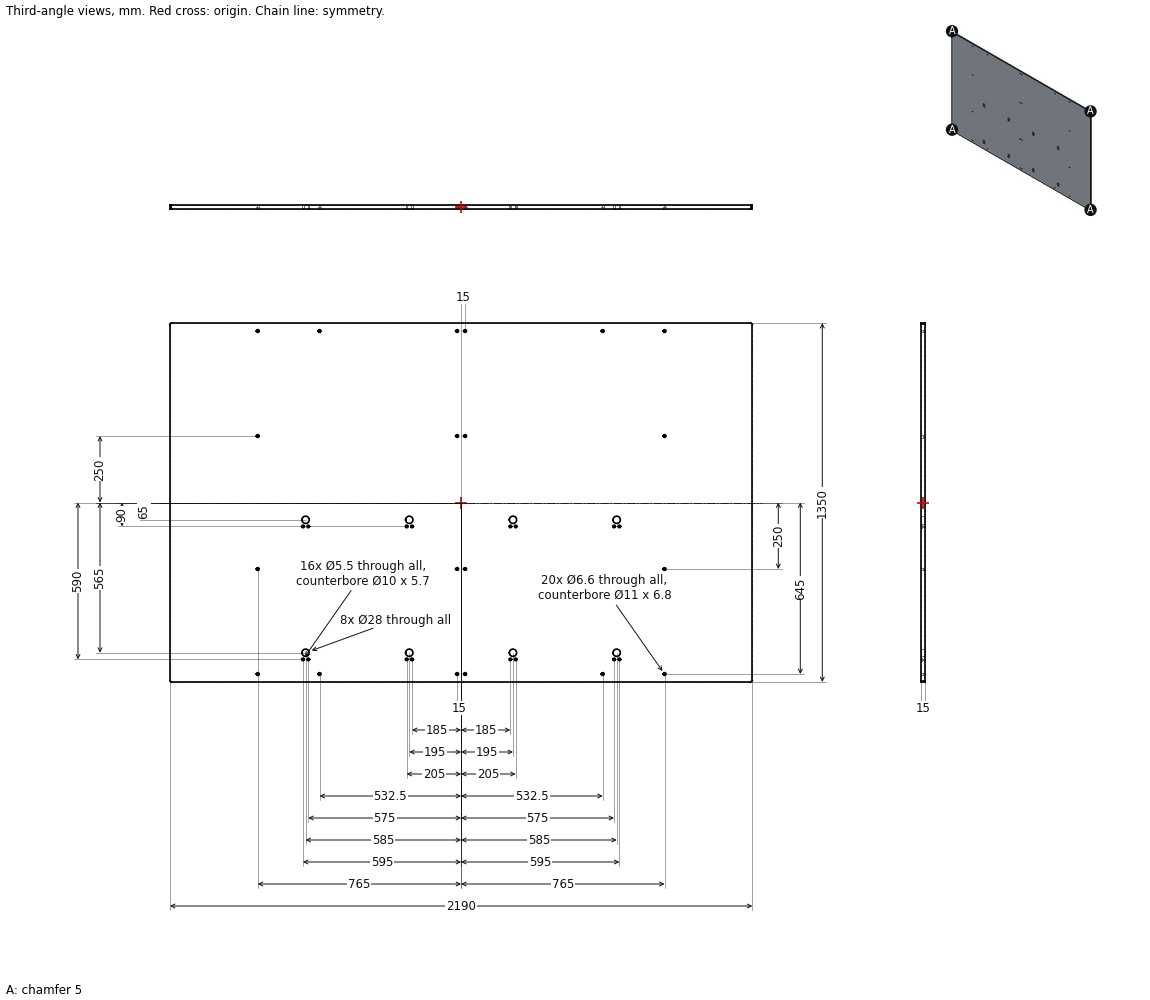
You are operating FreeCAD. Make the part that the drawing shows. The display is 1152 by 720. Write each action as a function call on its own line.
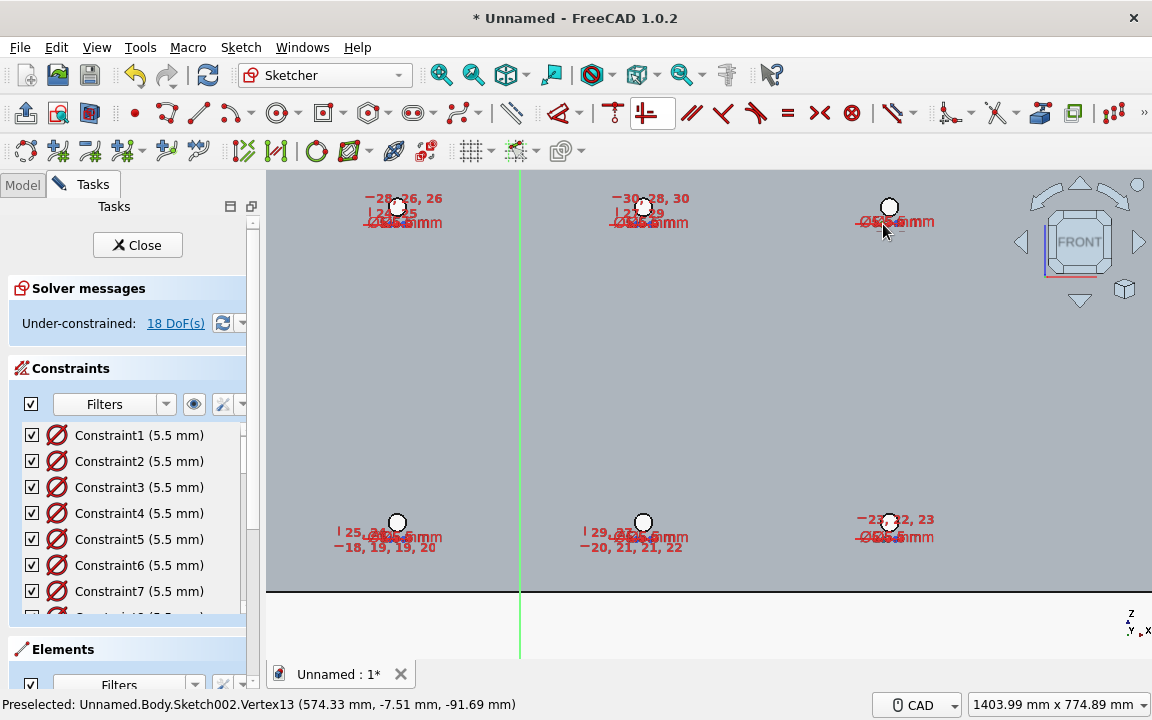
key(v)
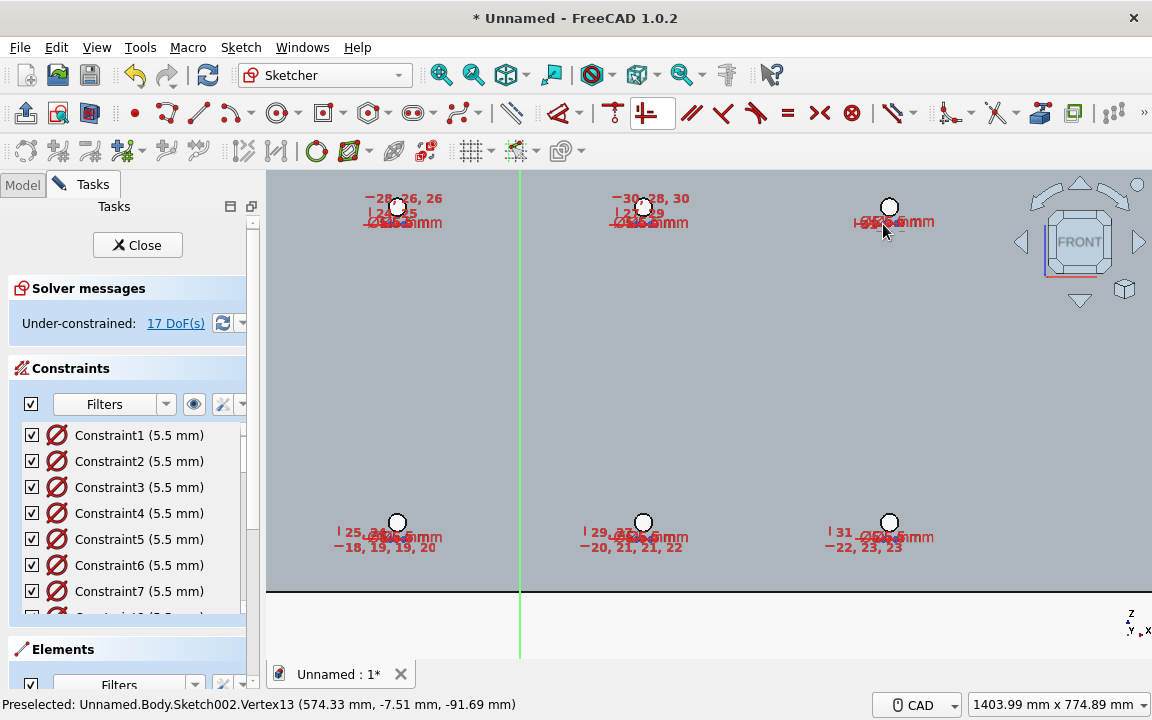
click(650, 225)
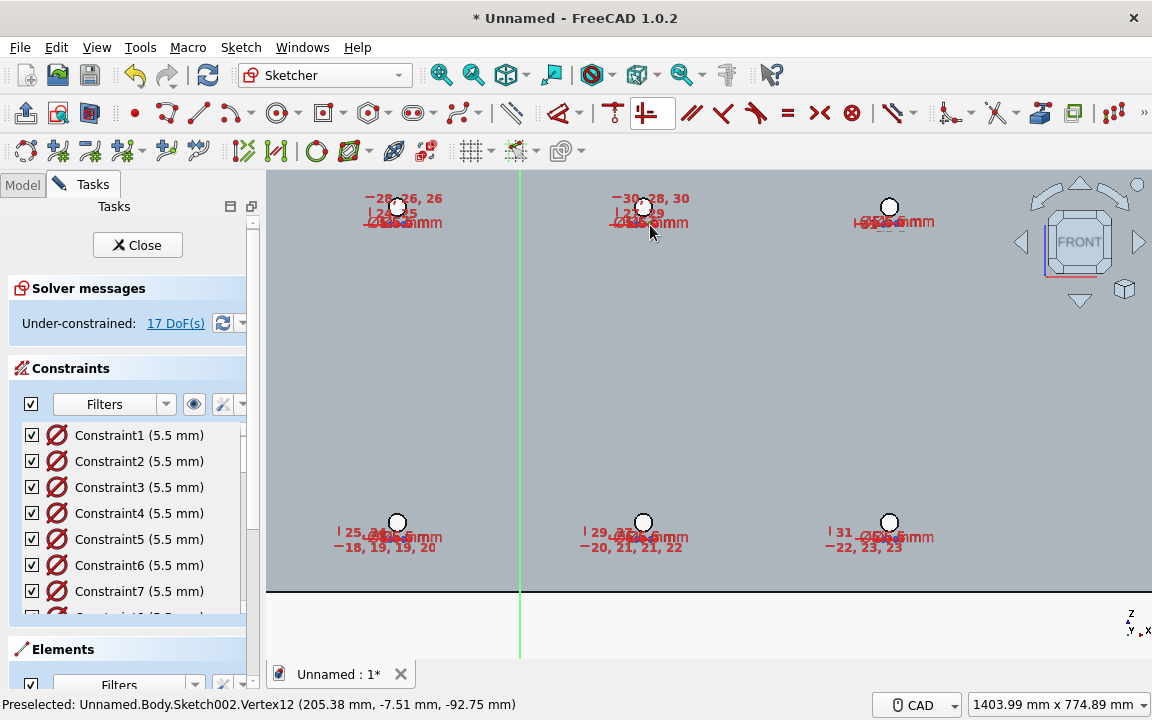
click(883, 224)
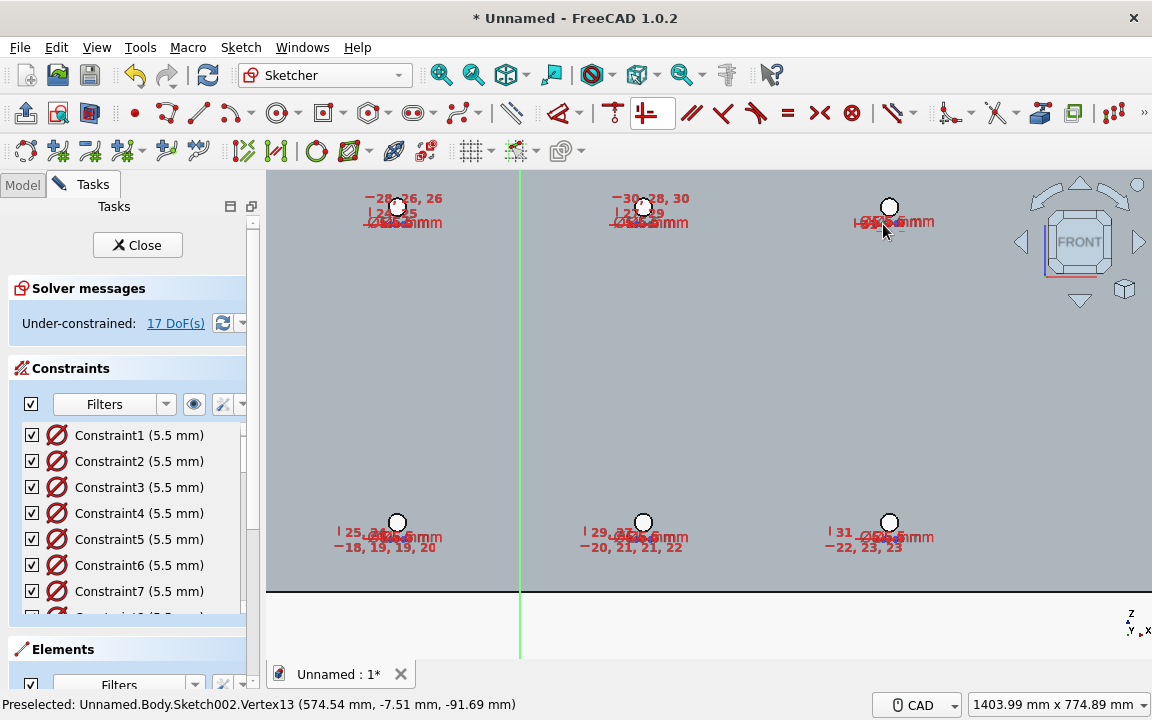
key(h)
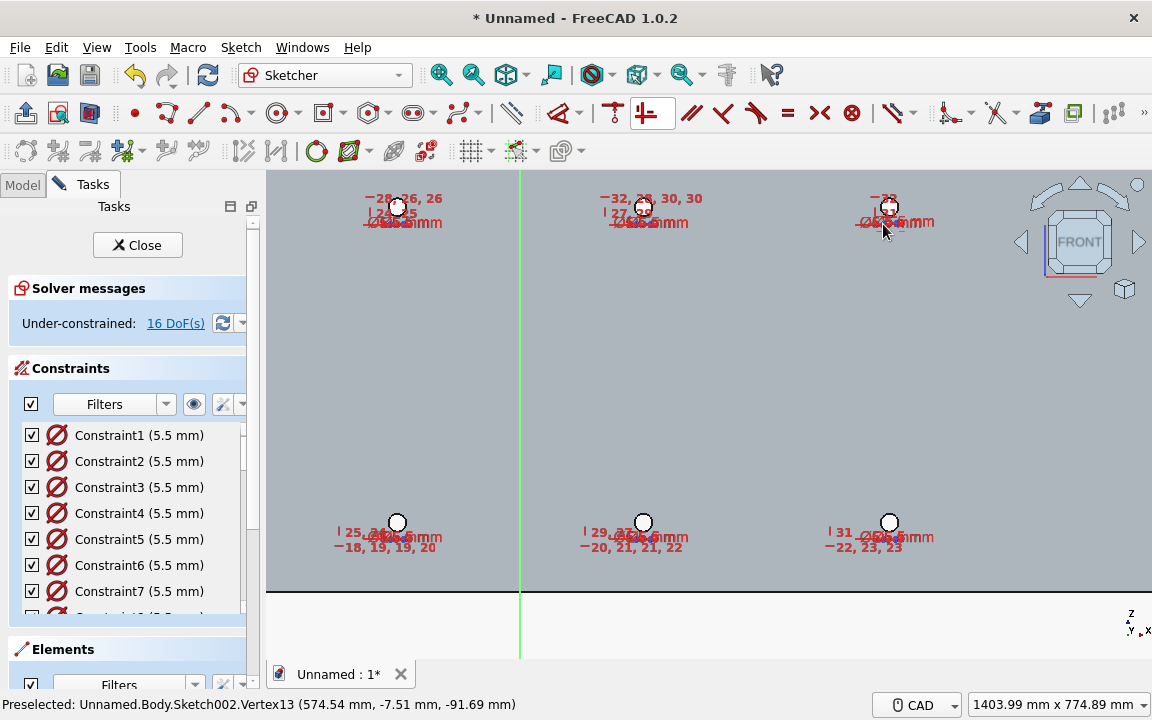
click(896, 539)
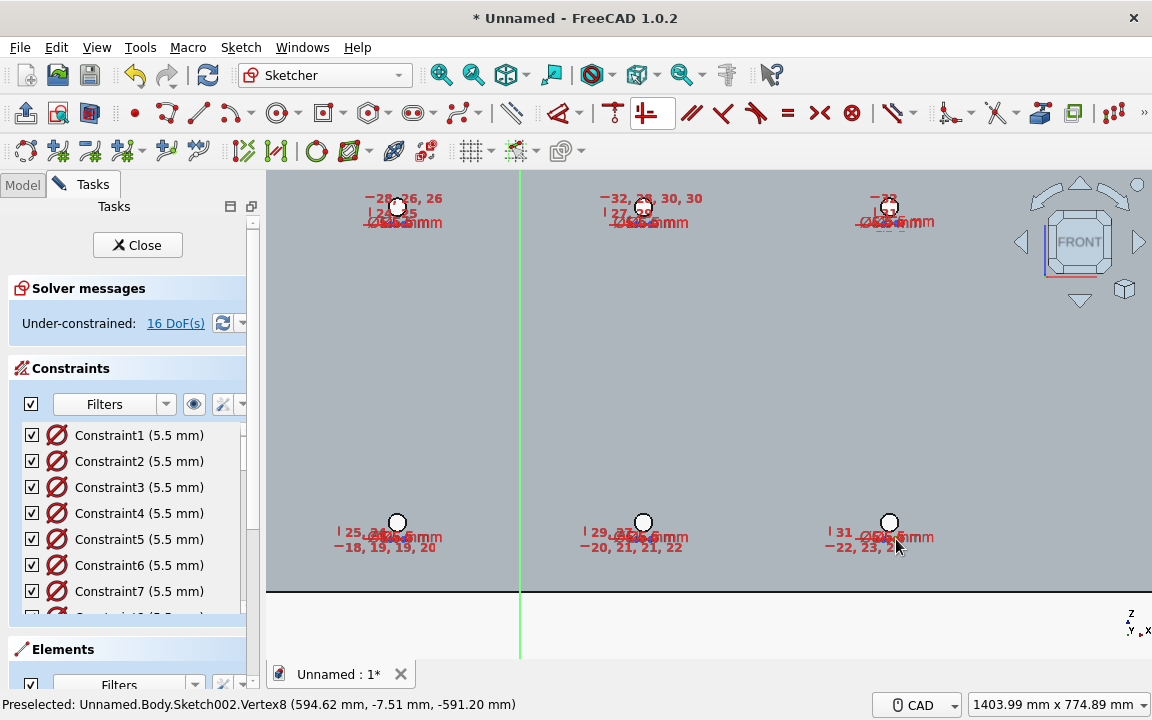
click(896, 224)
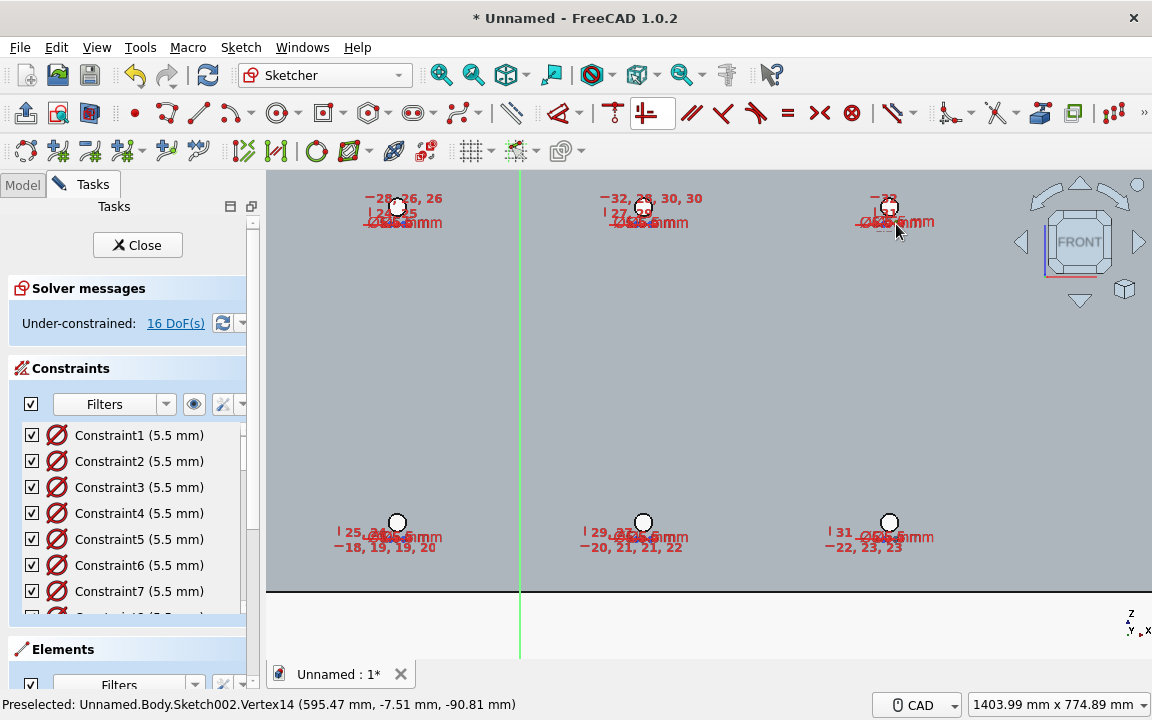
key(v)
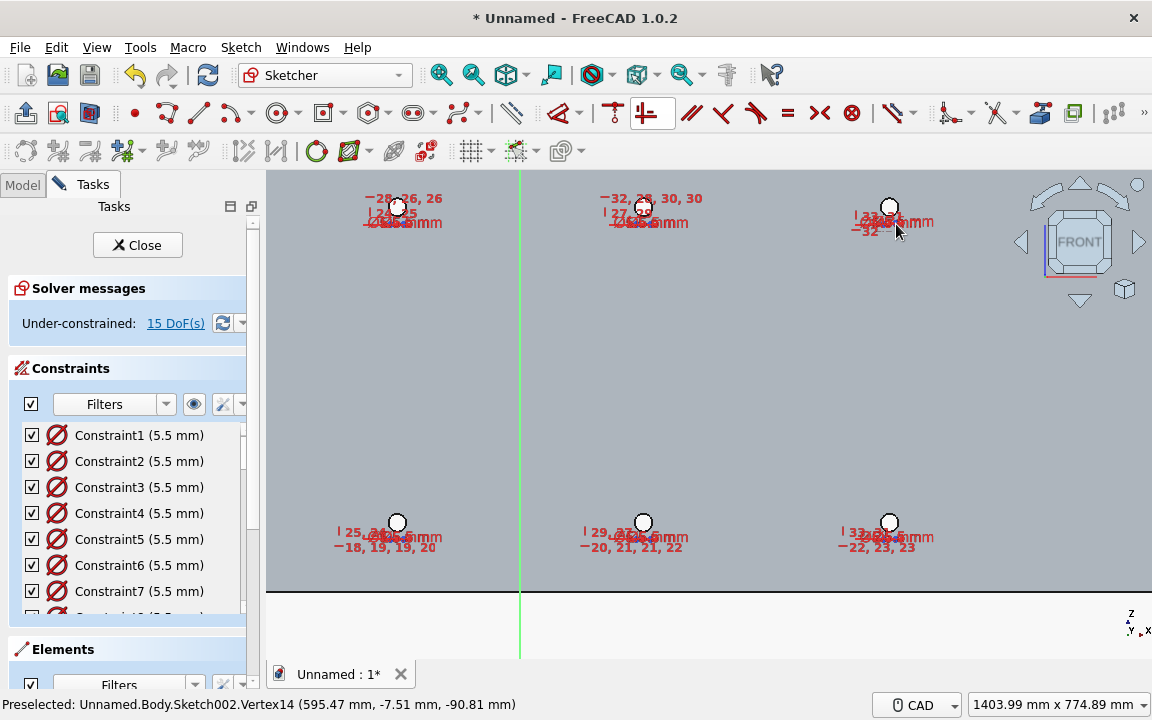
scroll(883, 225, up, 4)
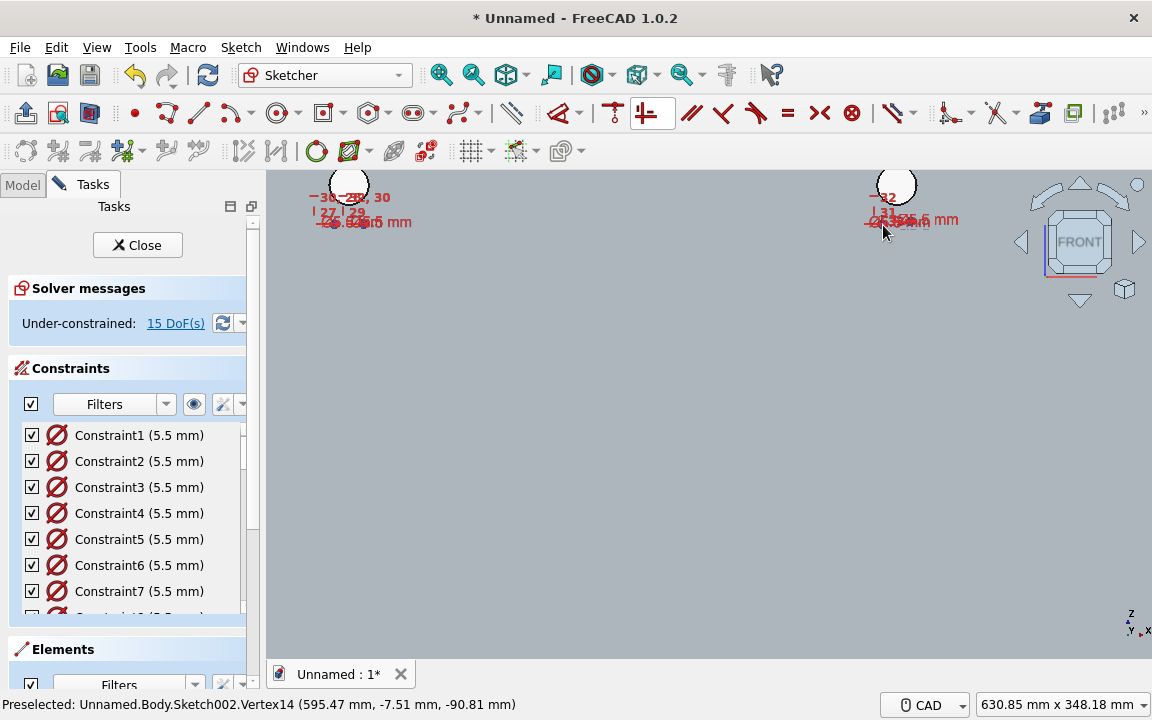
scroll(882, 224, up, 4)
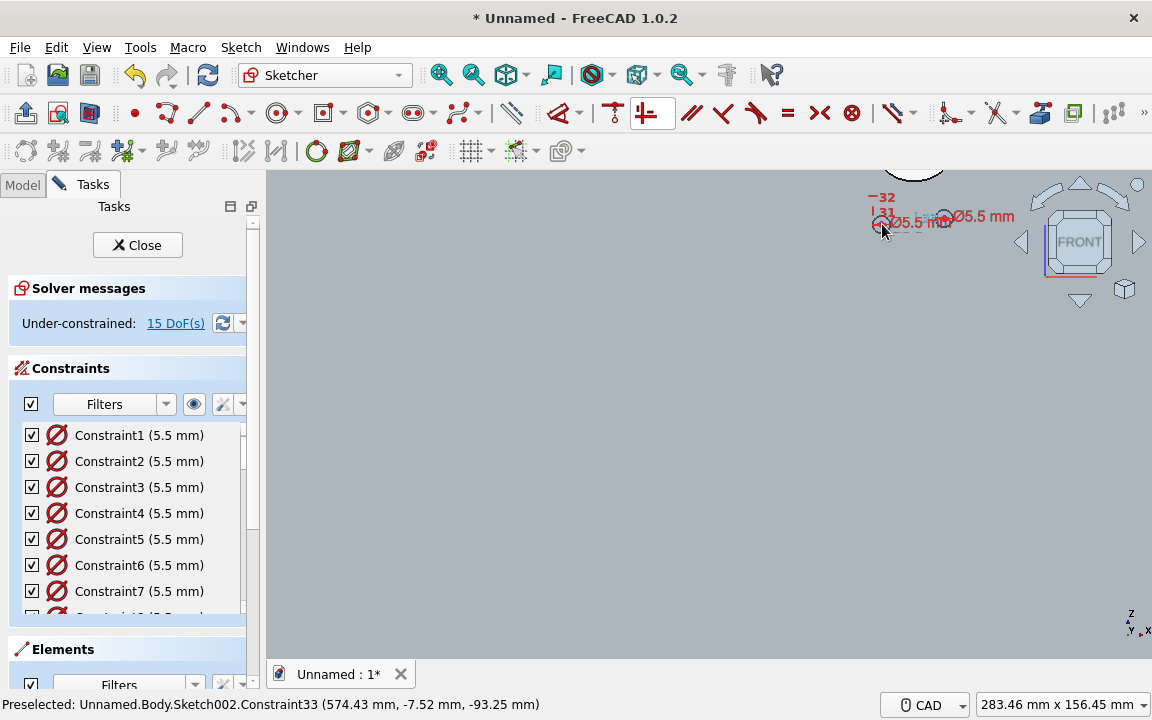
click(882, 225)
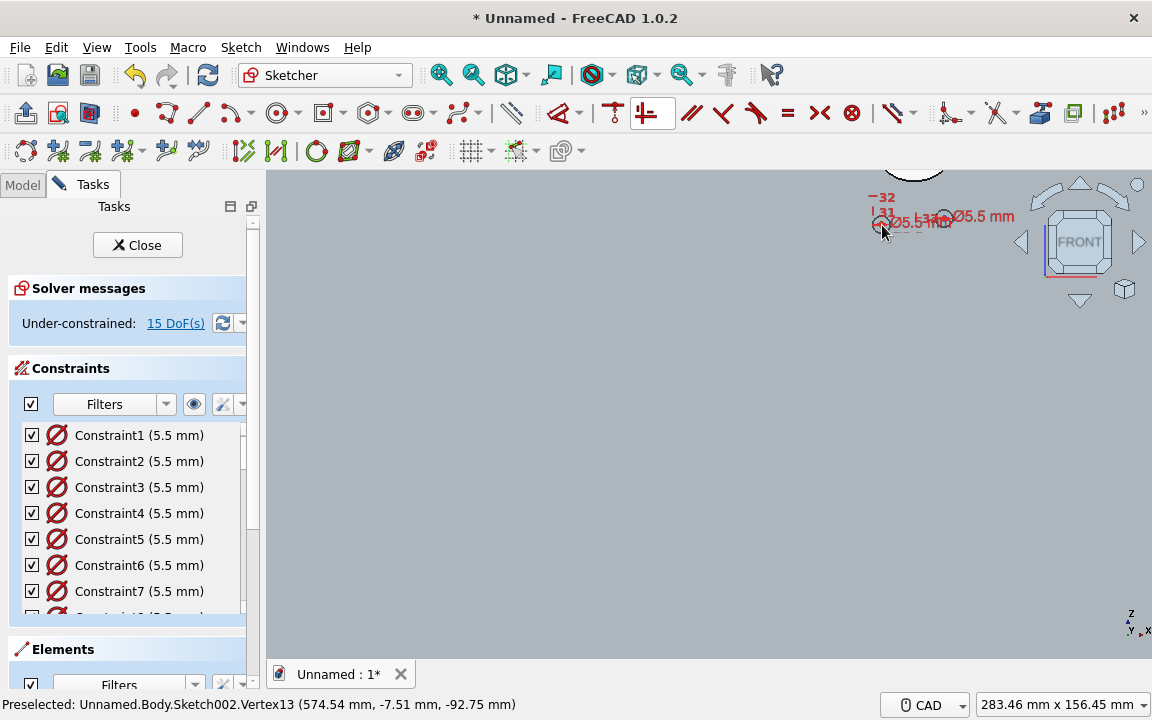
scroll(884, 345, down, 10)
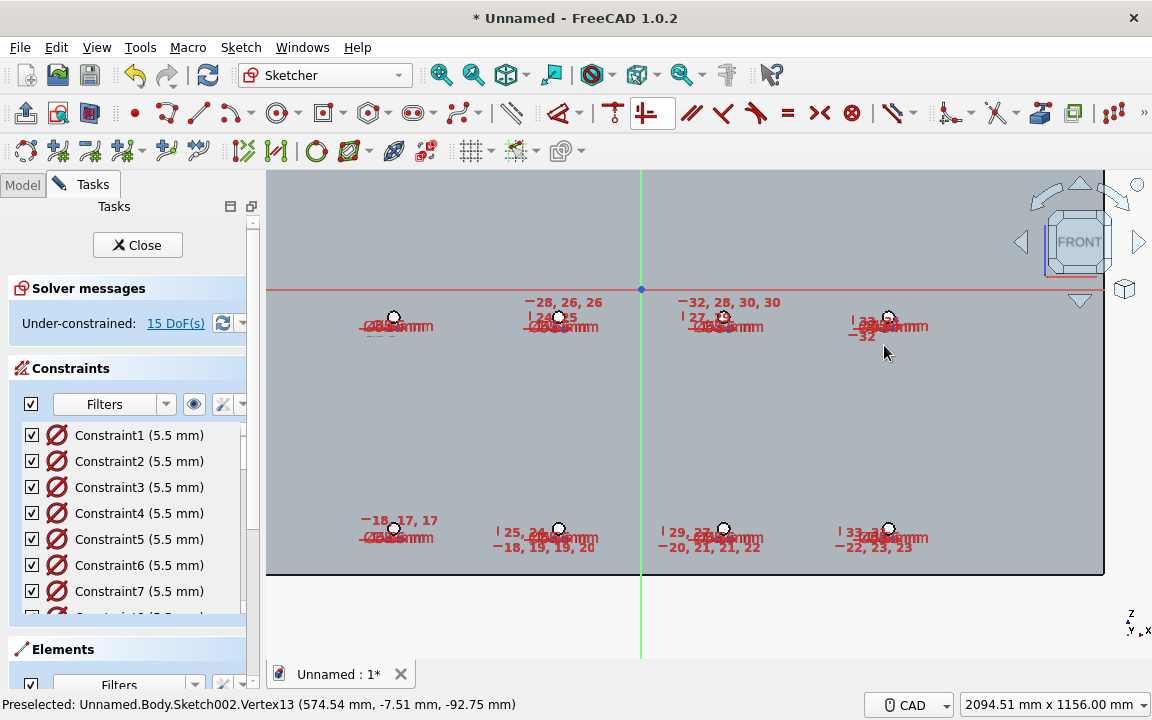
scroll(893, 328, up, 2)